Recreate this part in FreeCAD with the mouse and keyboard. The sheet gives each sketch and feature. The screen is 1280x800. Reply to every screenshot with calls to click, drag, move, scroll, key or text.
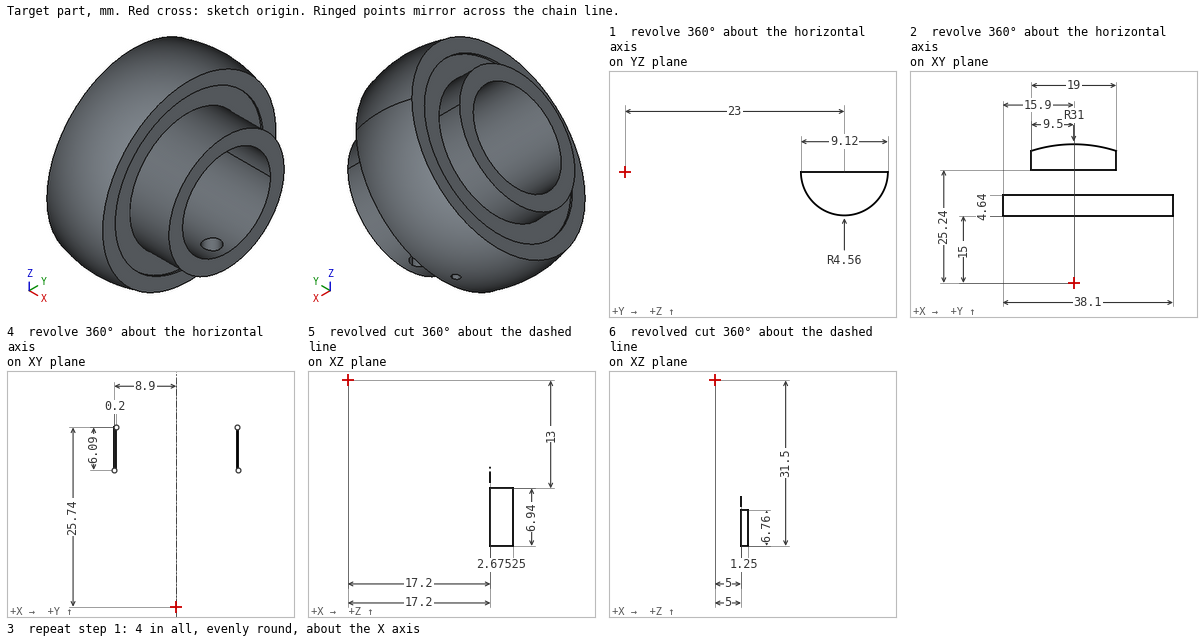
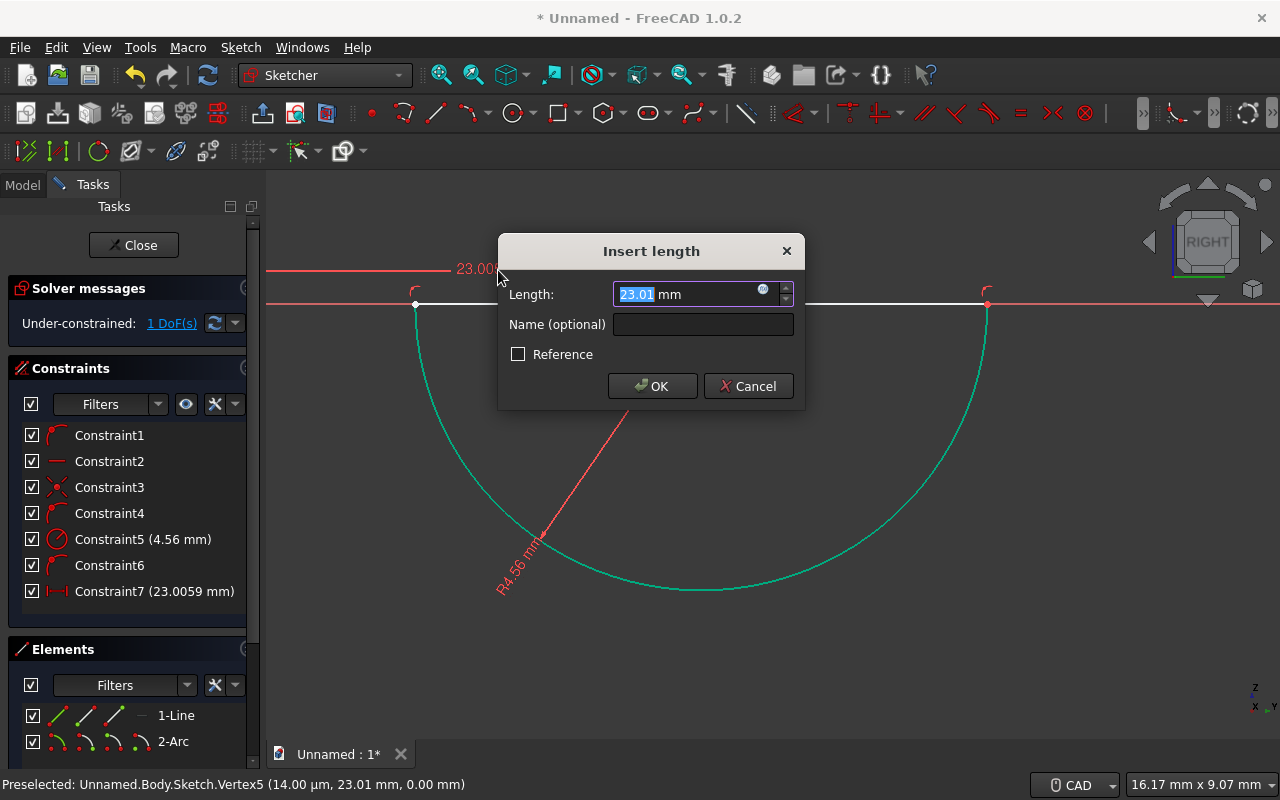
text(23)
key(Return)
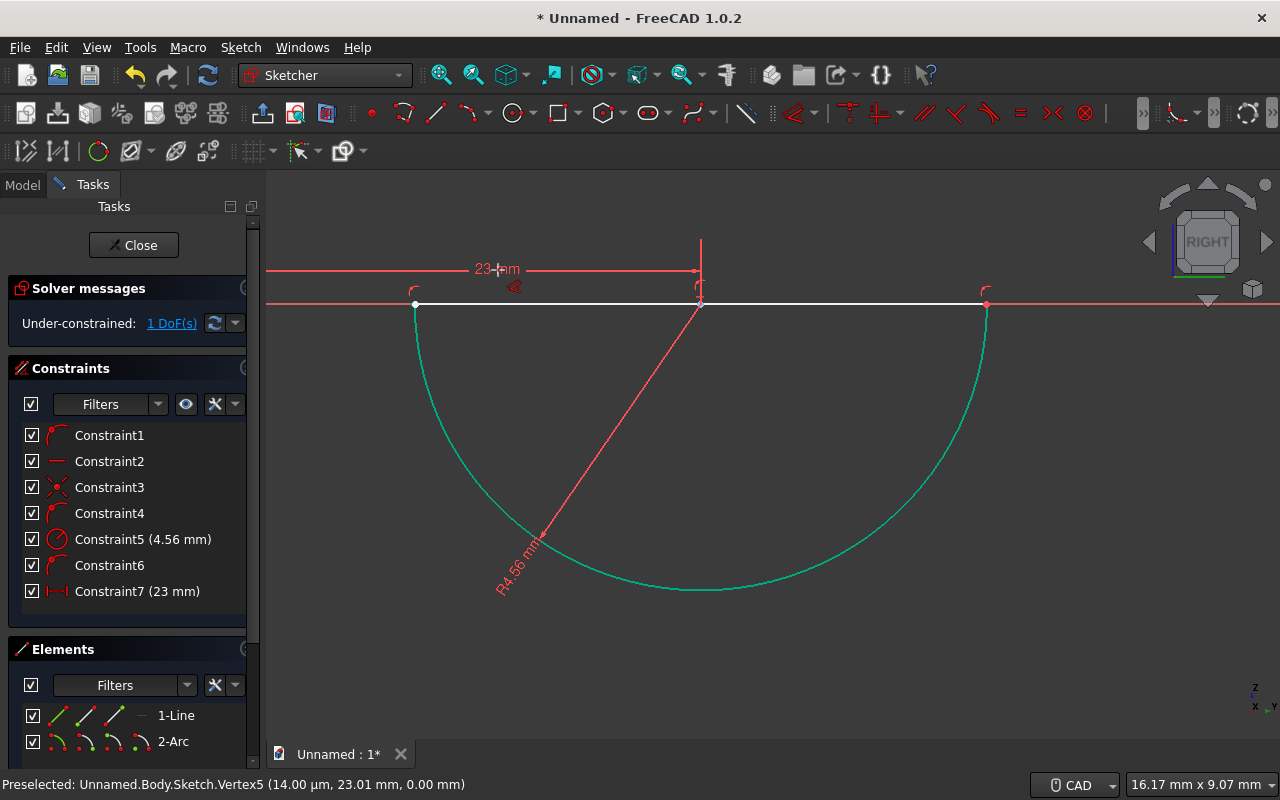
click(815, 304)
click(701, 270)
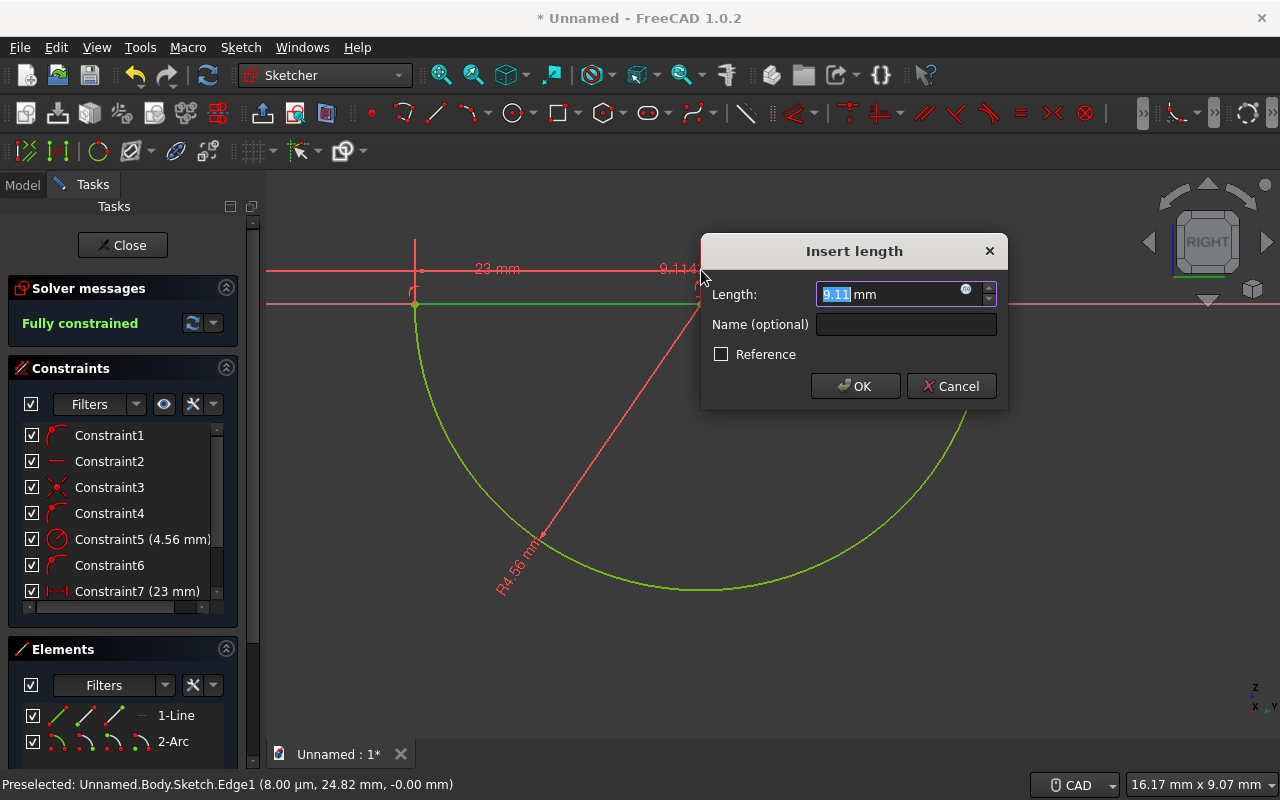
text(9.12)
key(Return)
key(Escape)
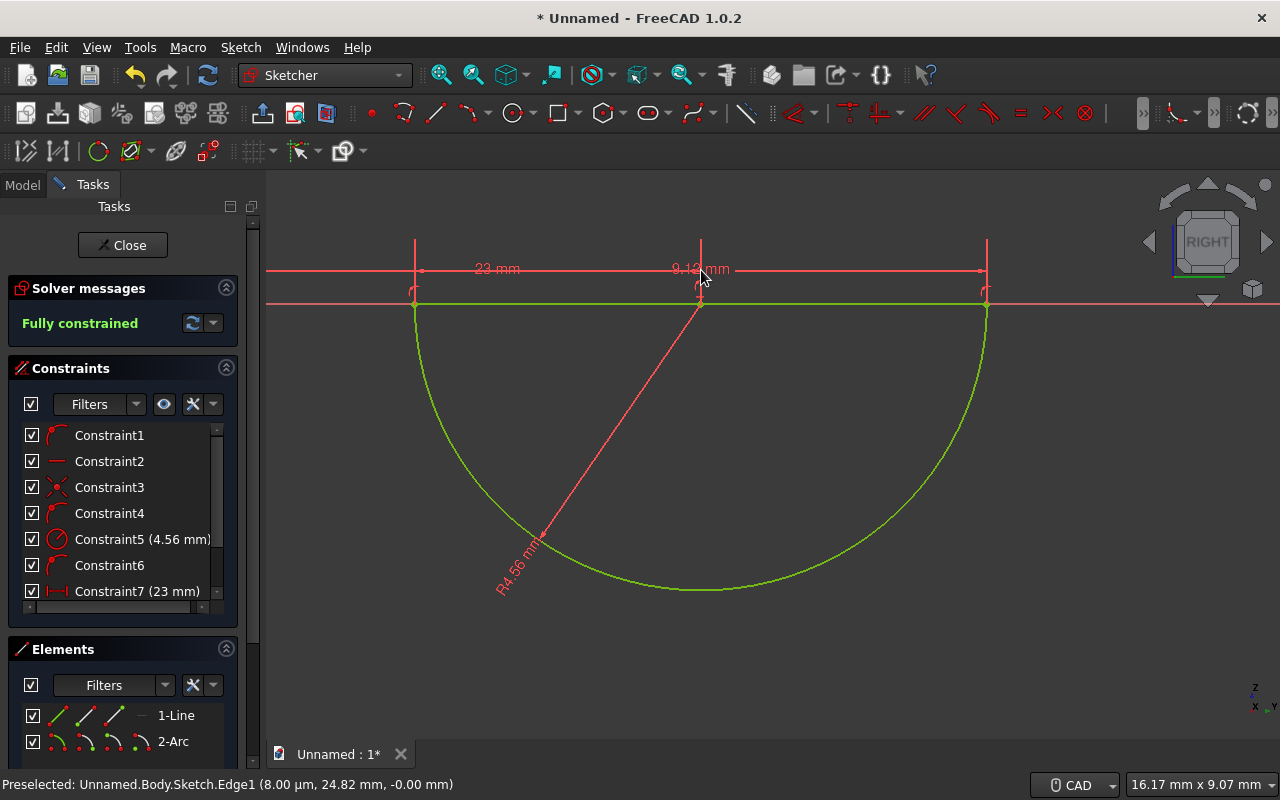
click(123, 245)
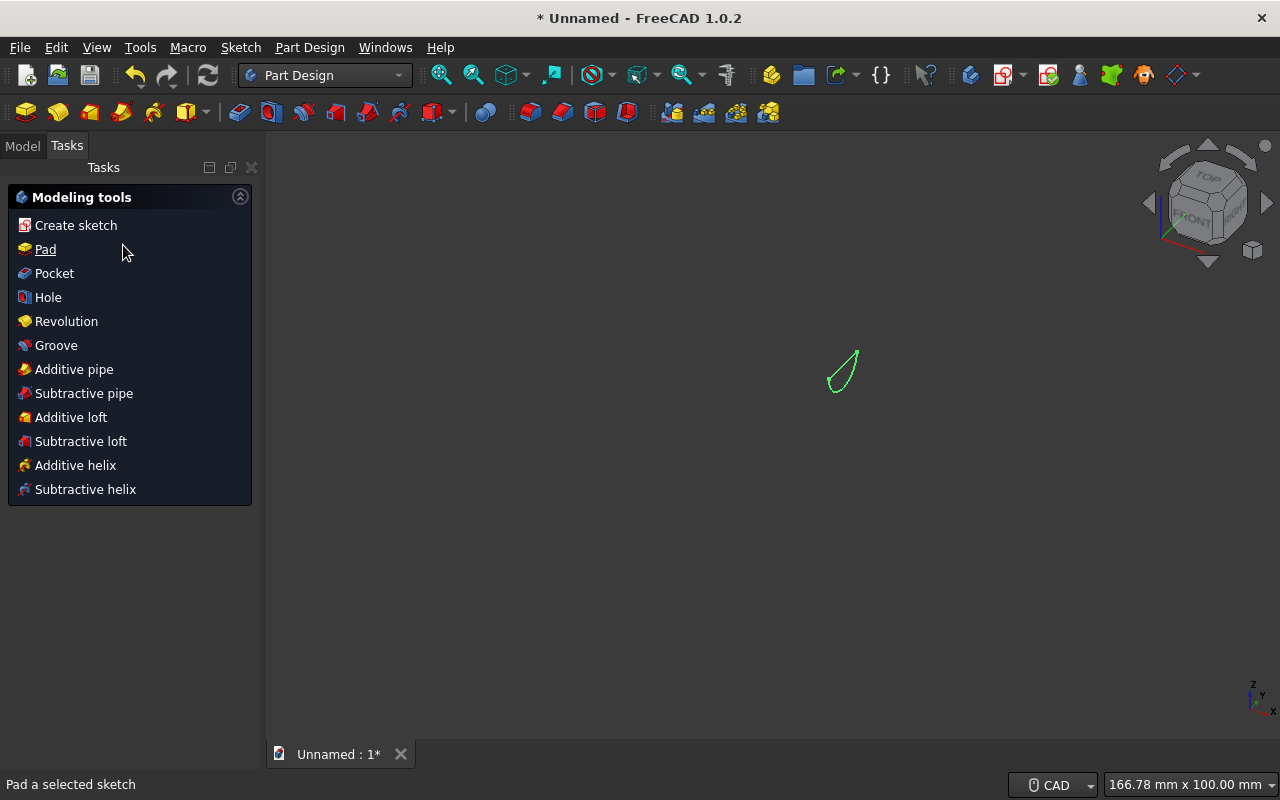
click(58, 112)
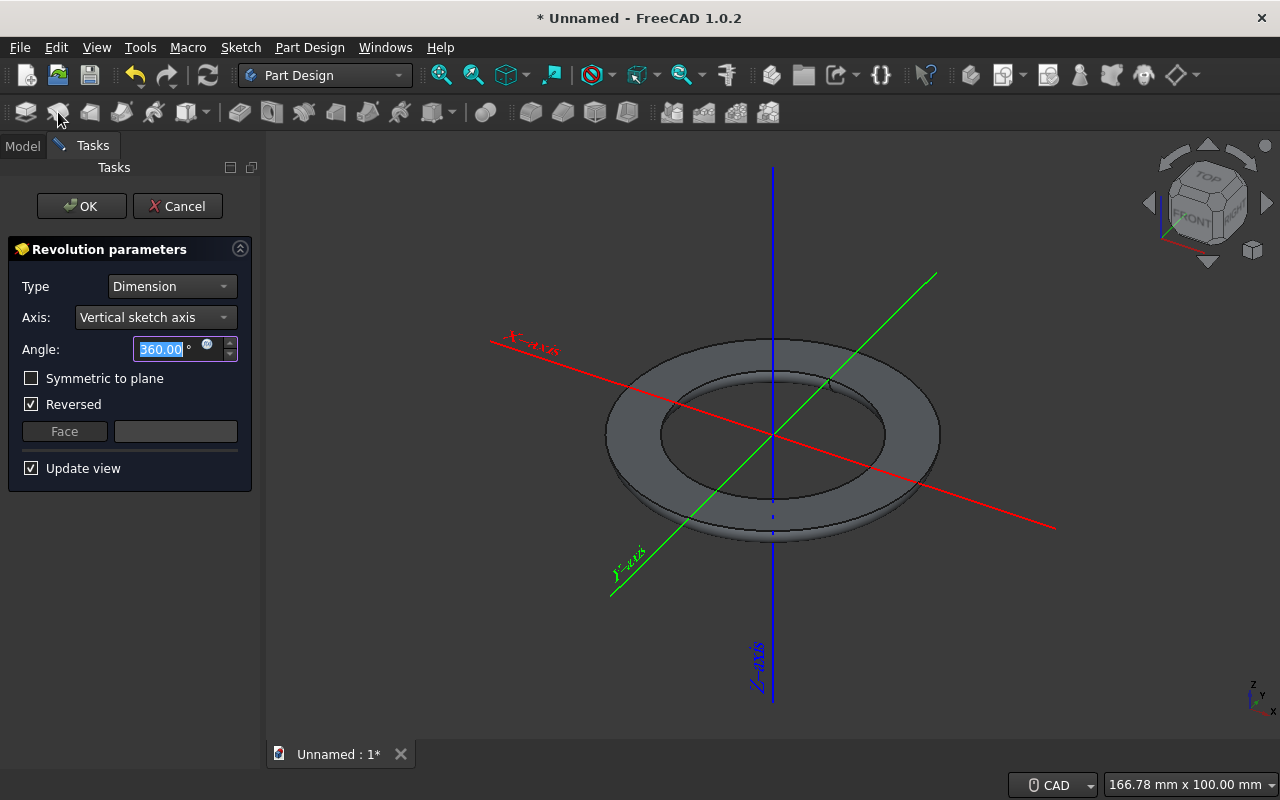
click(156, 318)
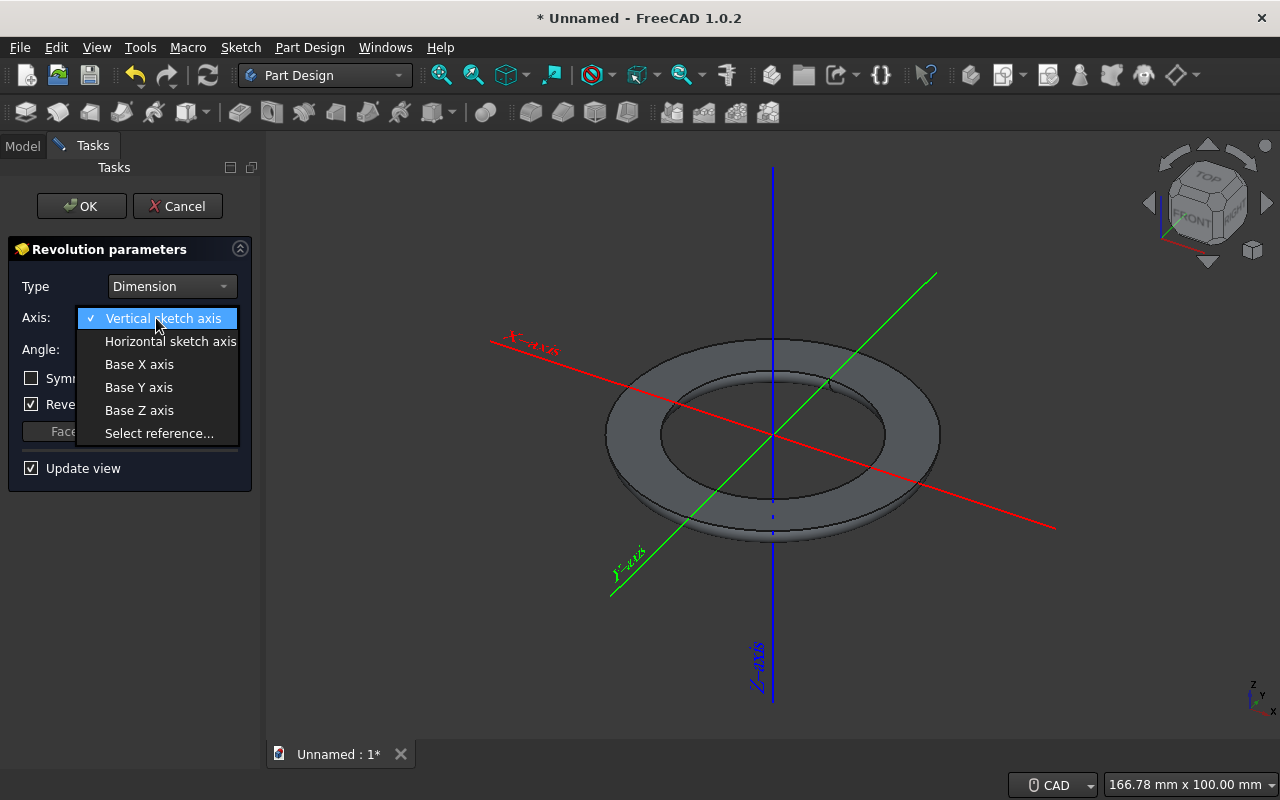
click(156, 342)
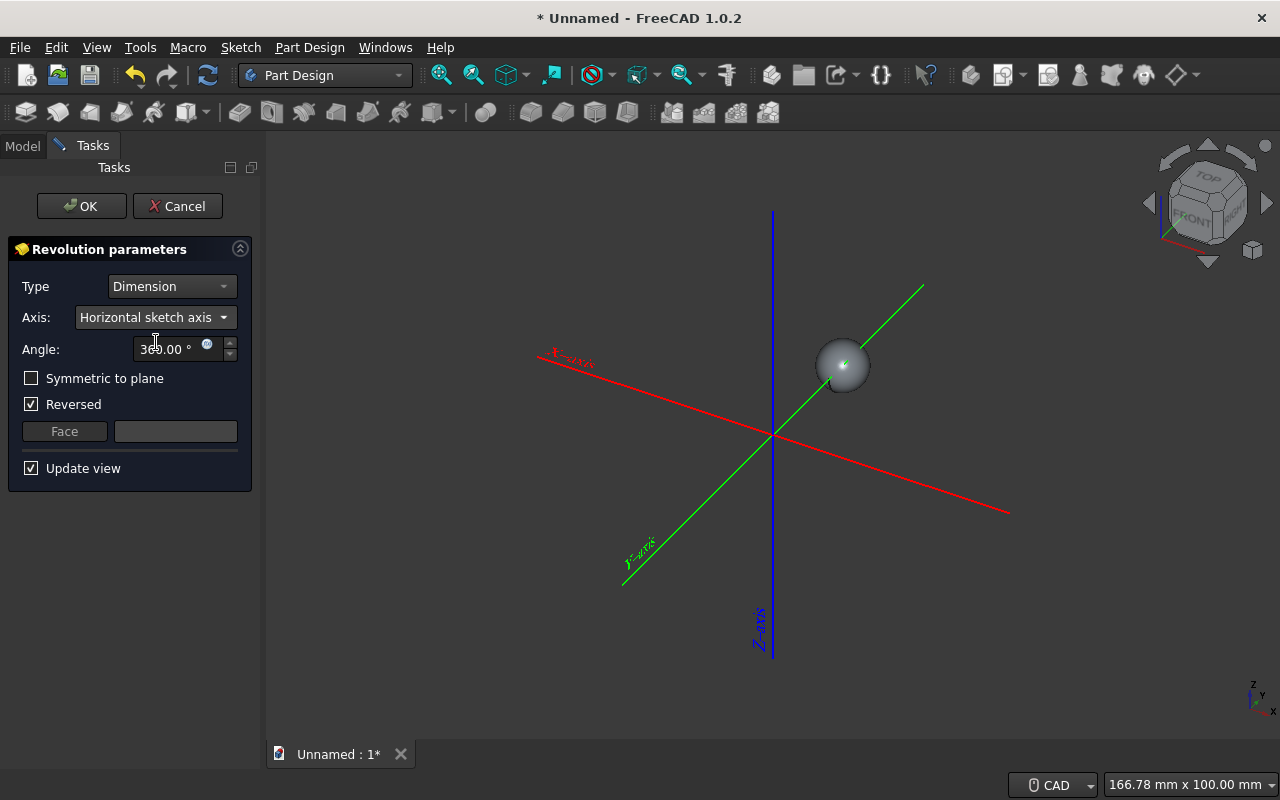
click(82, 206)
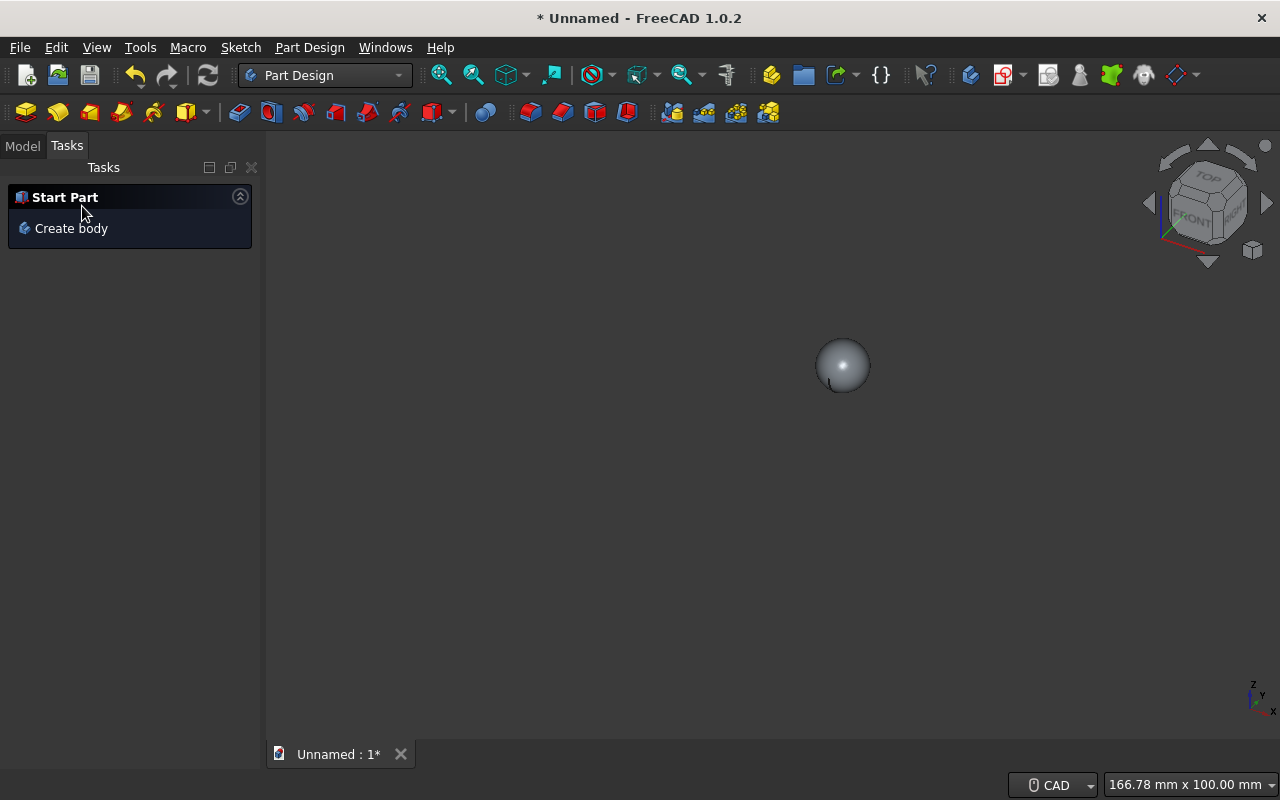
click(442, 76)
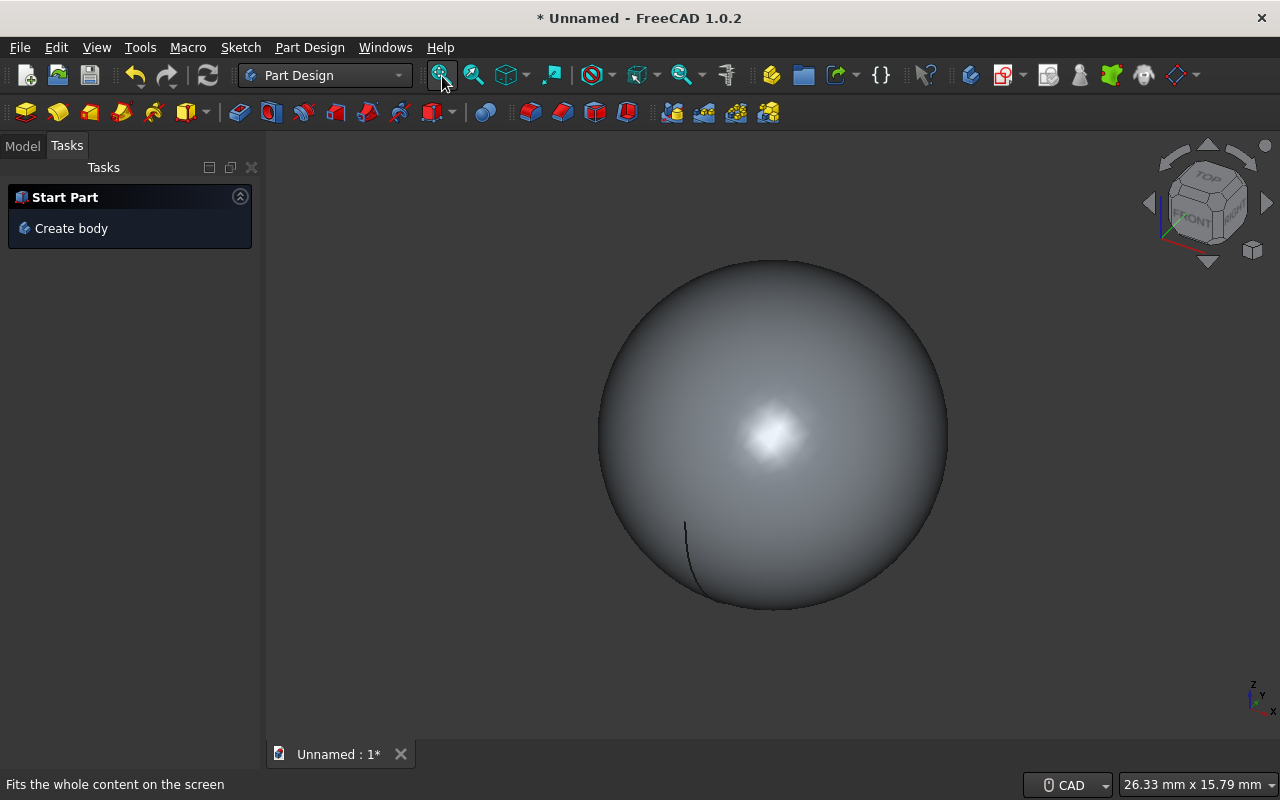
click(1004, 76)